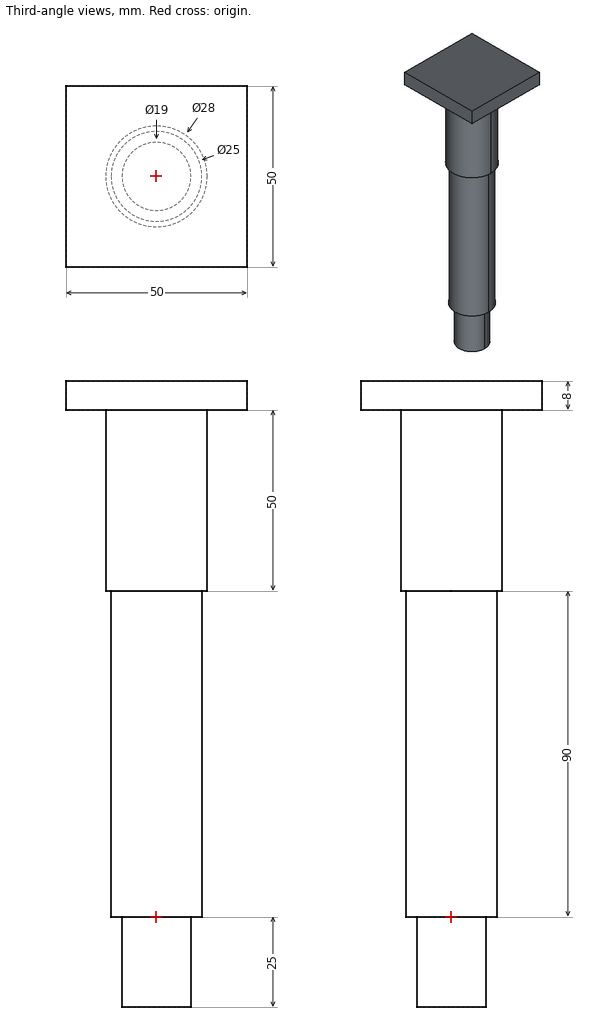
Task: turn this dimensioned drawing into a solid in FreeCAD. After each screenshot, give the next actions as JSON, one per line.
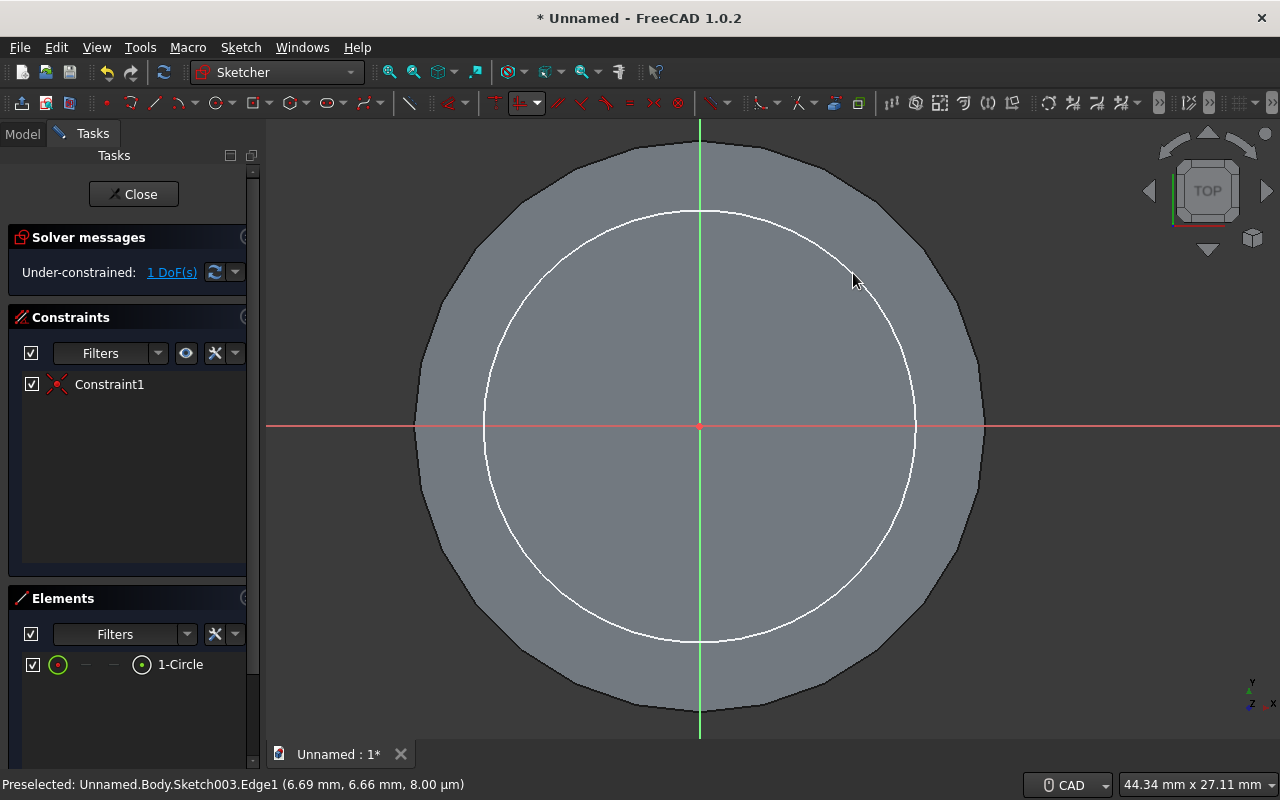
{"action": "left_click", "coordinate": [448, 104]}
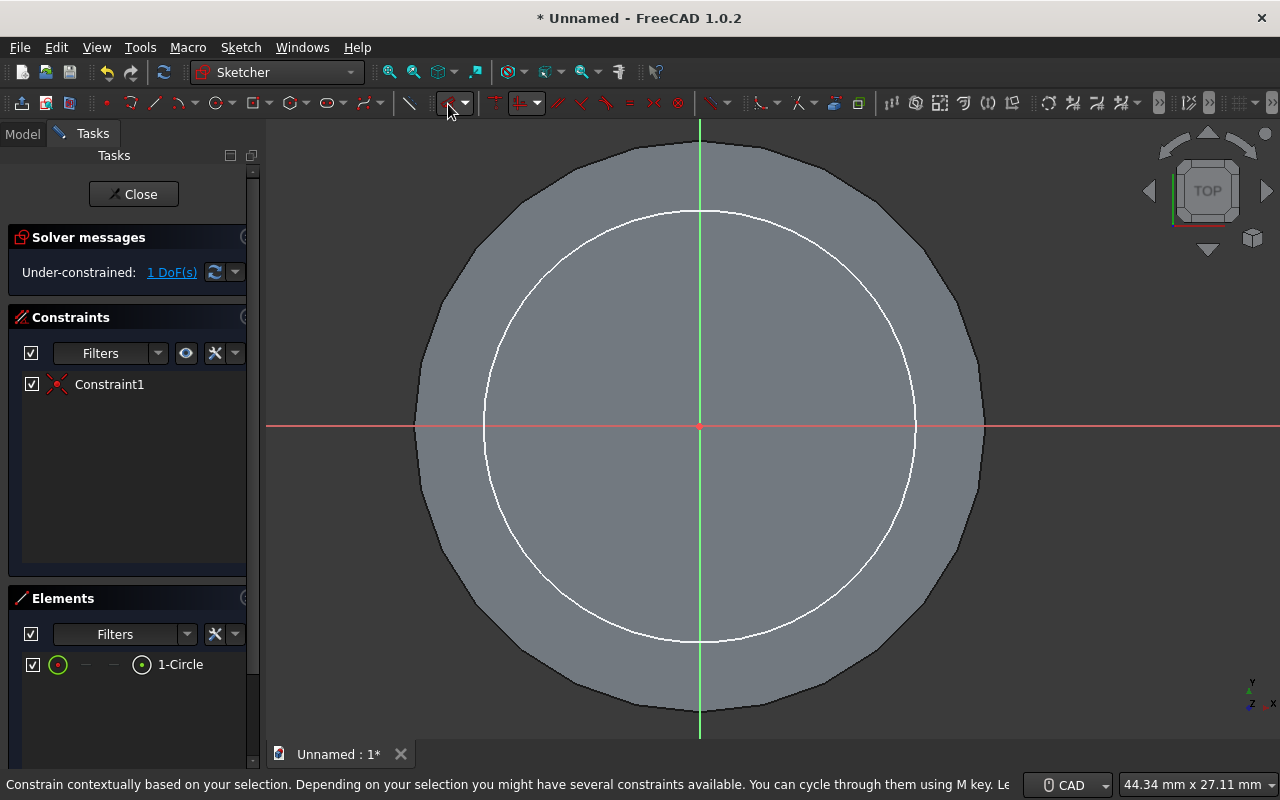
{"action": "left_click", "coordinate": [852, 273]}
{"action": "left_click", "coordinate": [875, 250]}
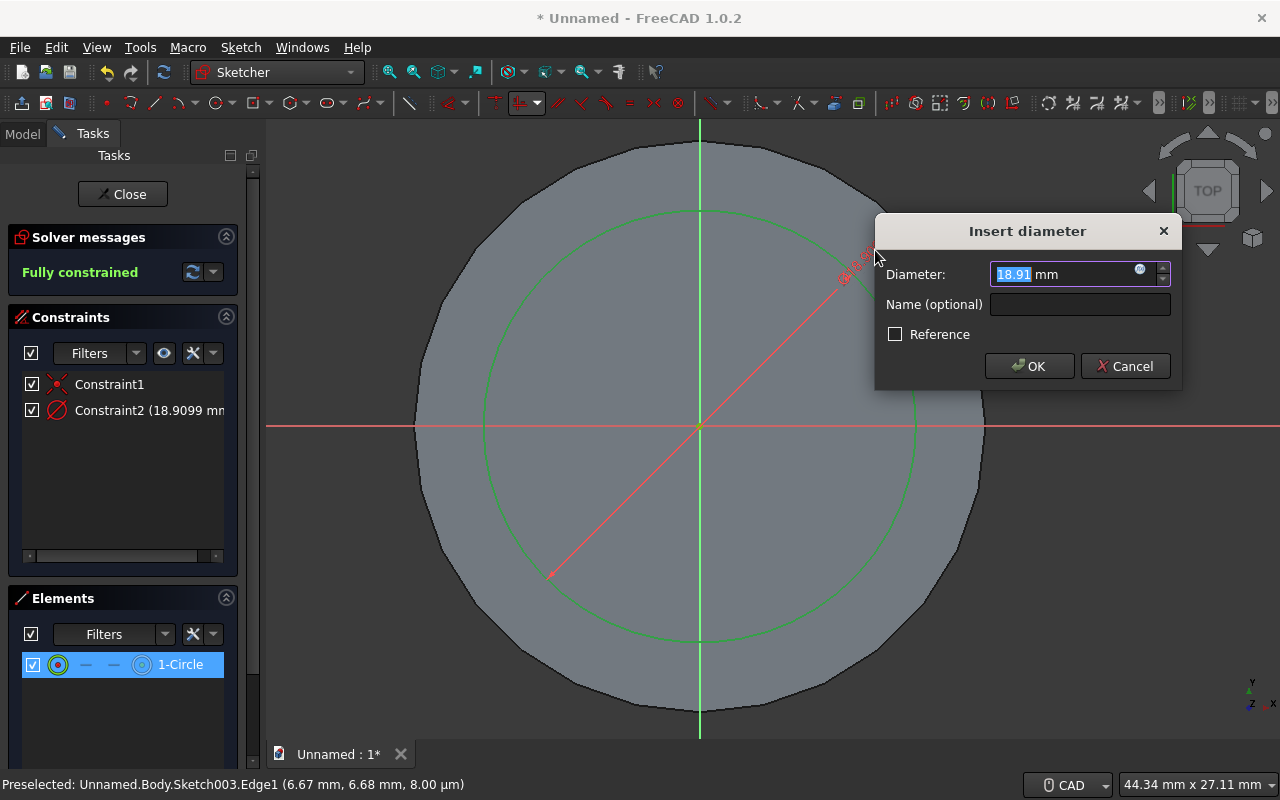
{"action": "type", "text": "19"}
{"action": "key", "text": "Return"}
{"action": "key", "text": "Escape"}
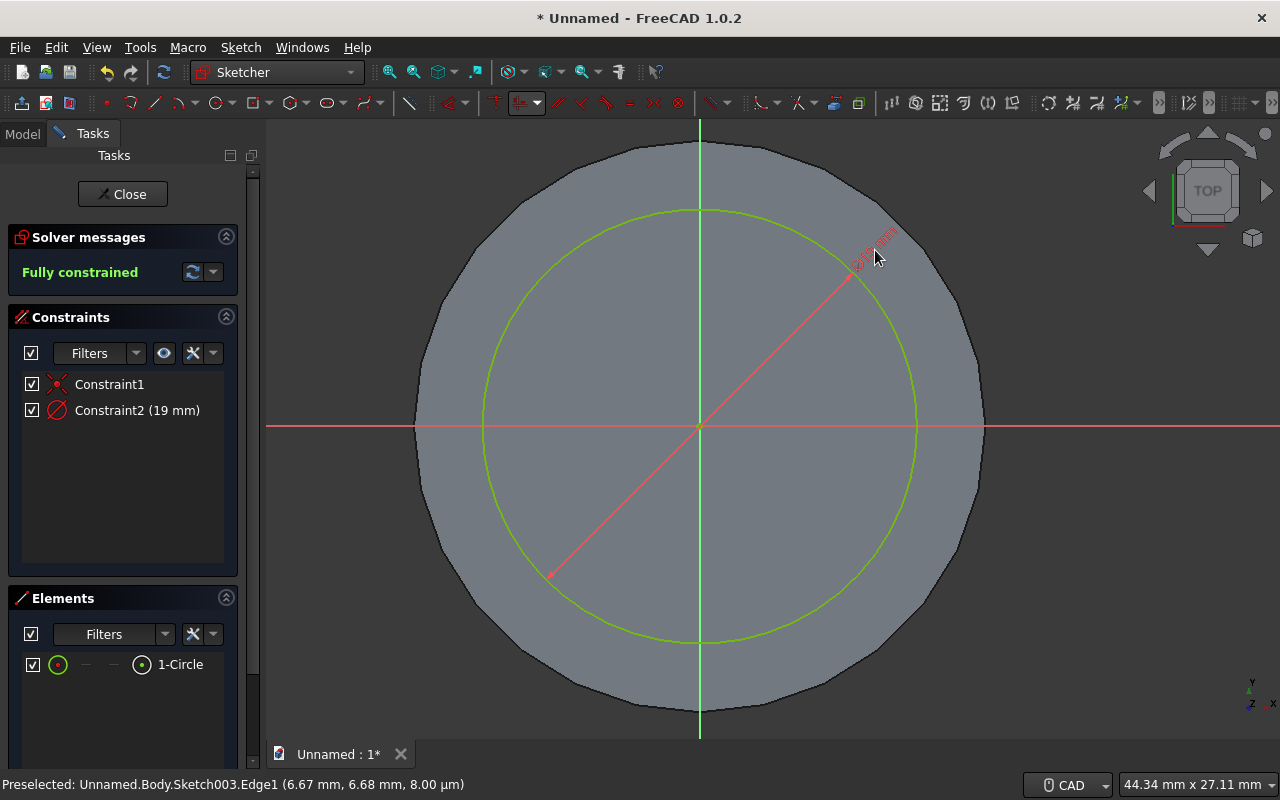
{"action": "left_click", "coordinate": [123, 194]}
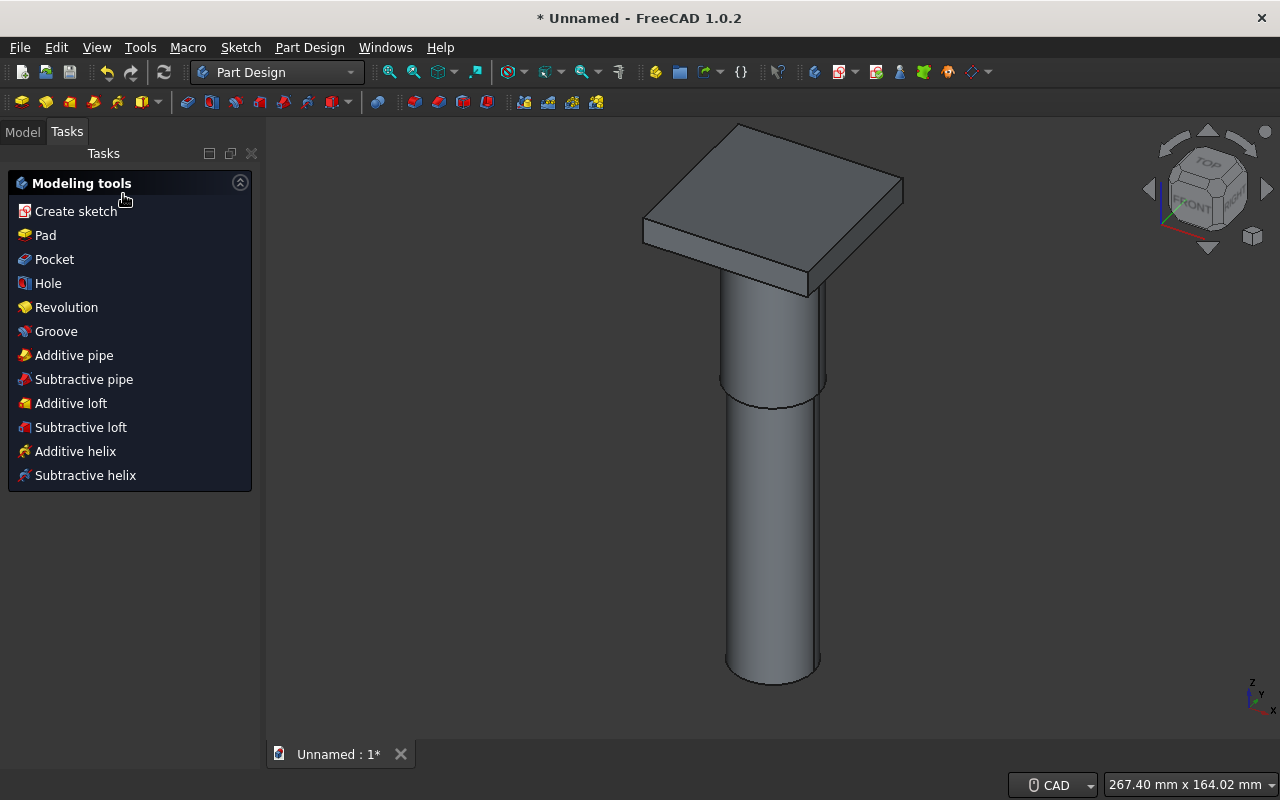
{"action": "left_click", "coordinate": [22, 102]}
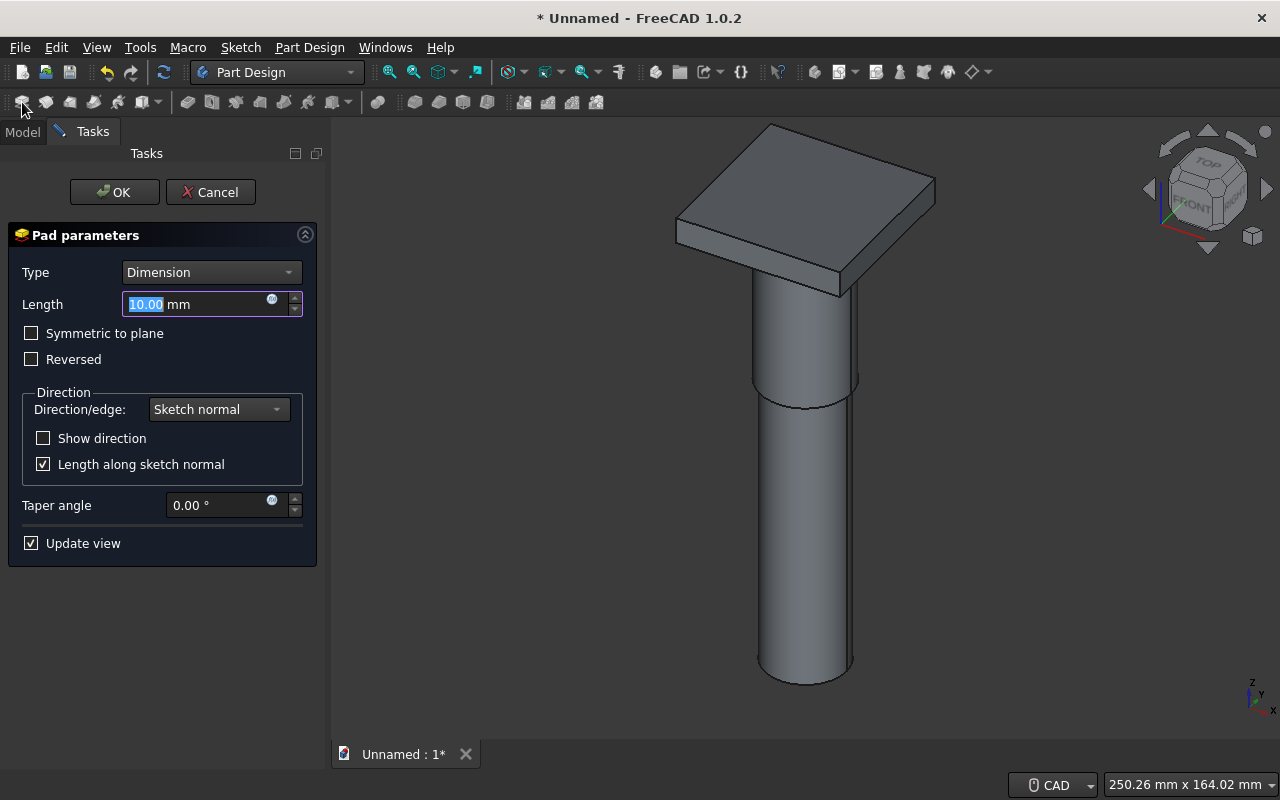
{"action": "type", "text": "25"}
{"action": "key", "text": "Tab"}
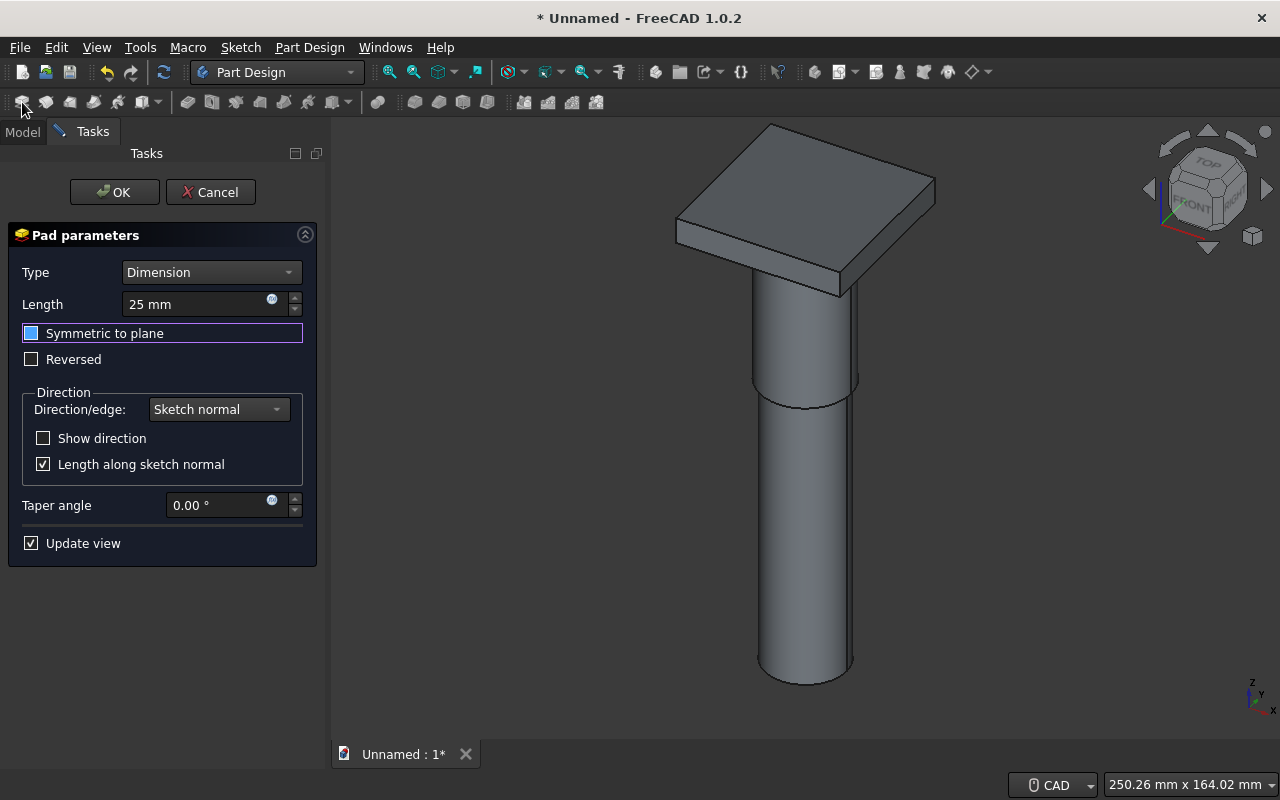
{"action": "left_click", "coordinate": [30, 359]}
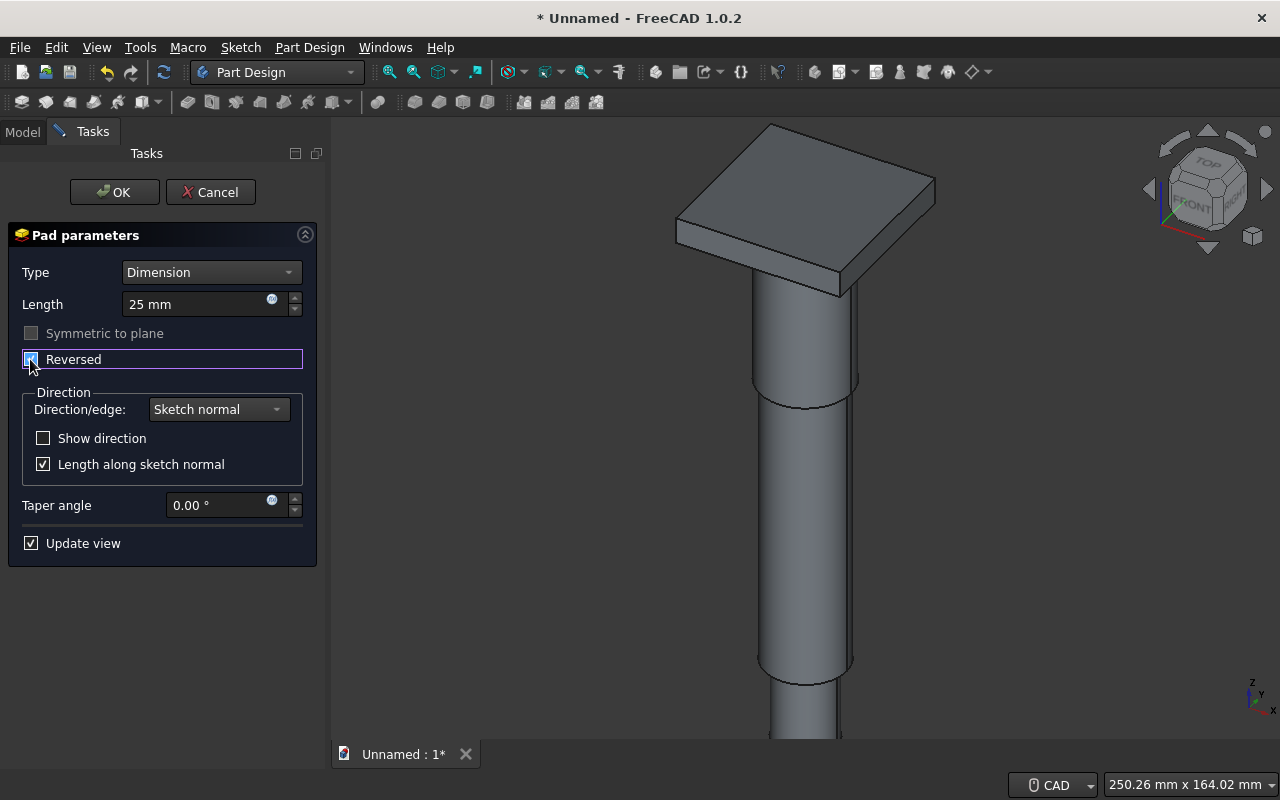
{"action": "left_click", "coordinate": [115, 192]}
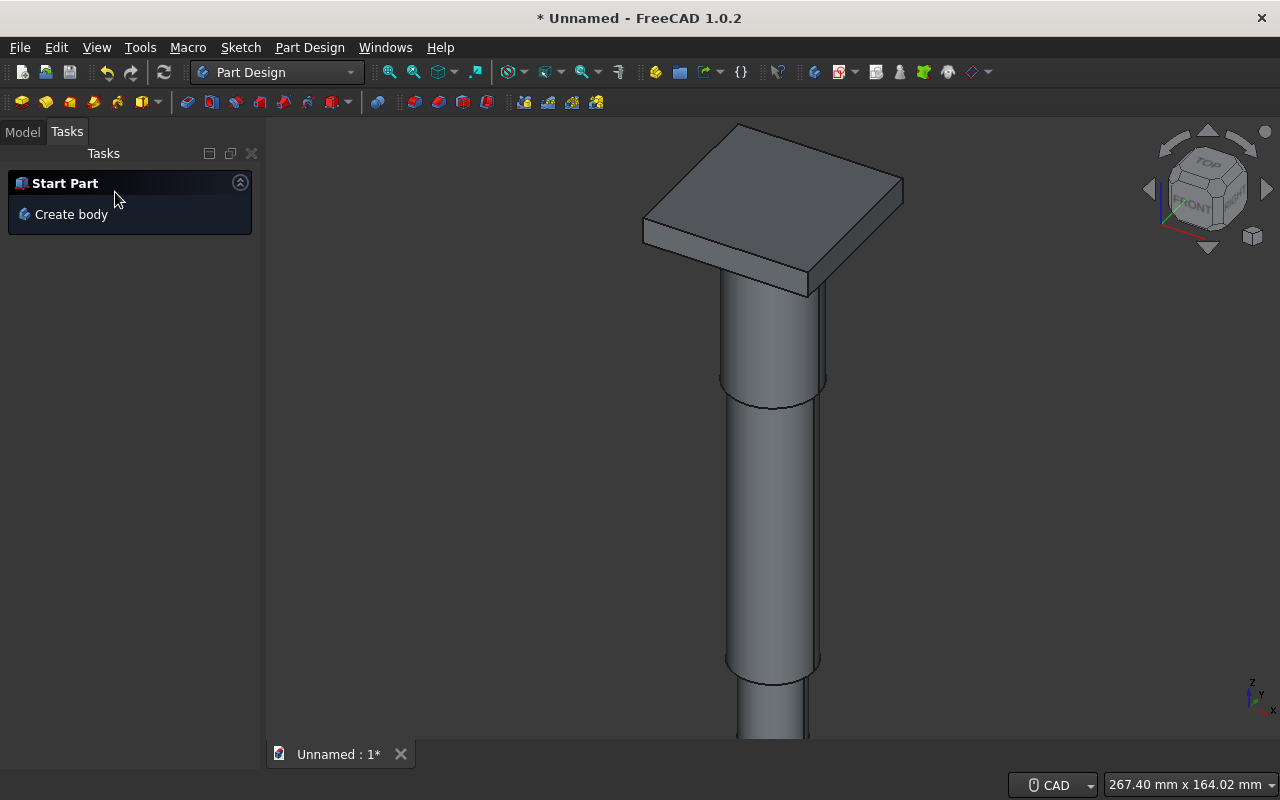
{"action": "key", "text": "0"}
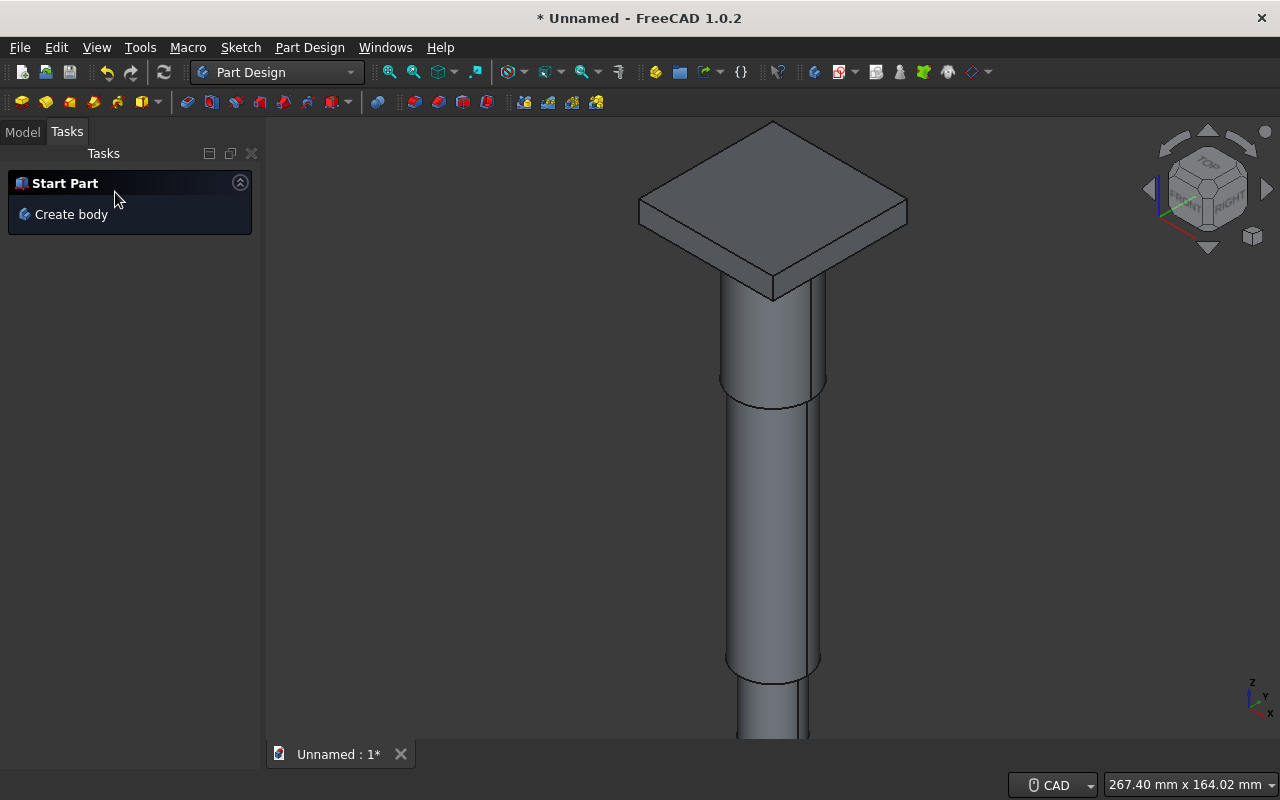
{"action": "key", "text": "v f"}